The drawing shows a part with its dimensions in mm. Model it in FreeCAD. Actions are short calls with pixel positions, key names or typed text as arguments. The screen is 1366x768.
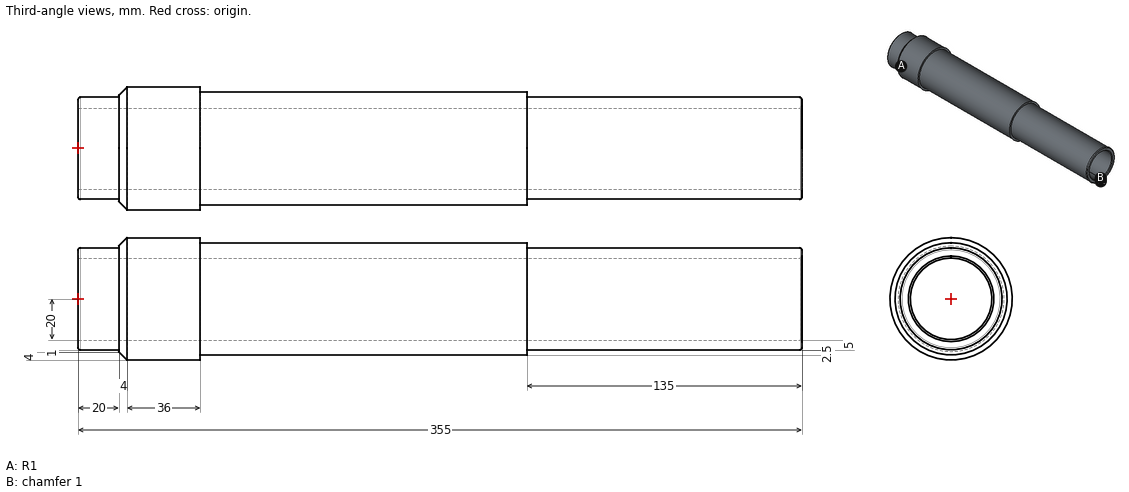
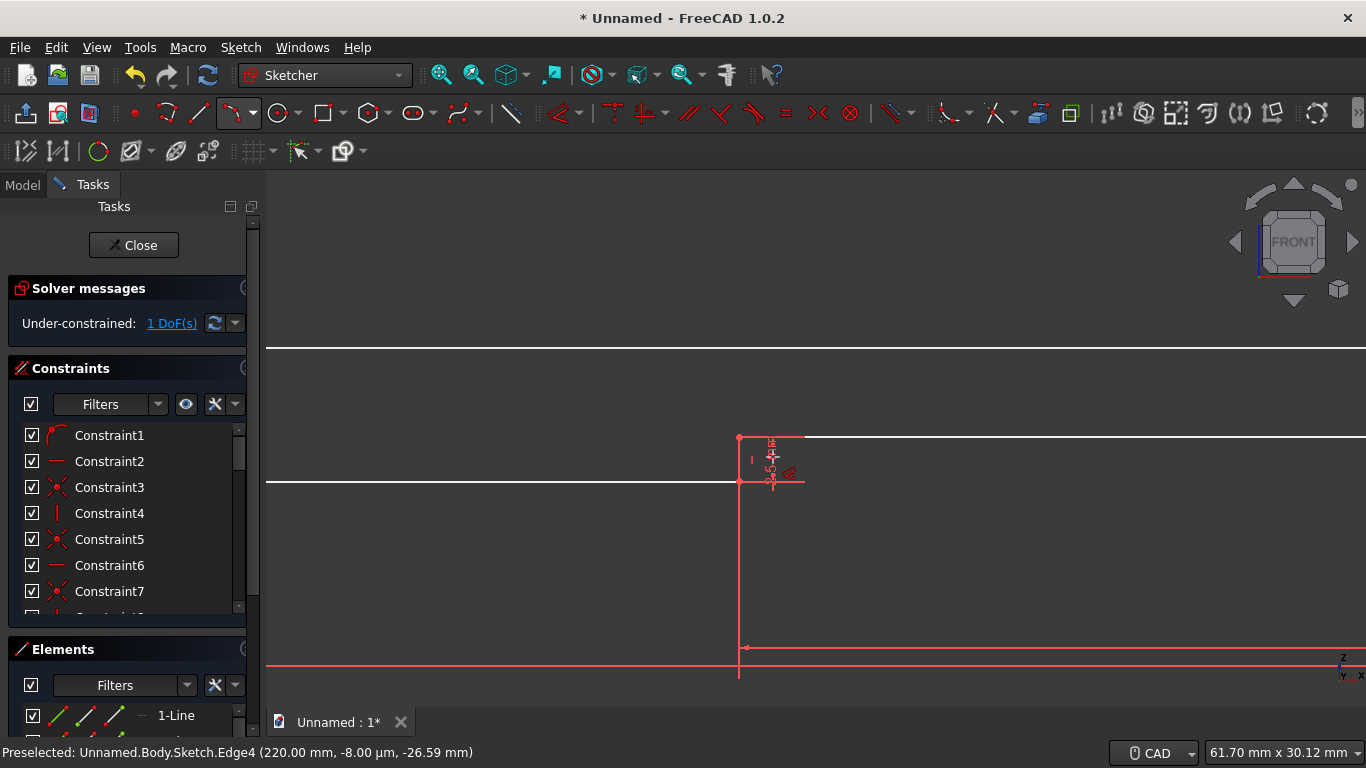
scroll(843, 462, down, 11)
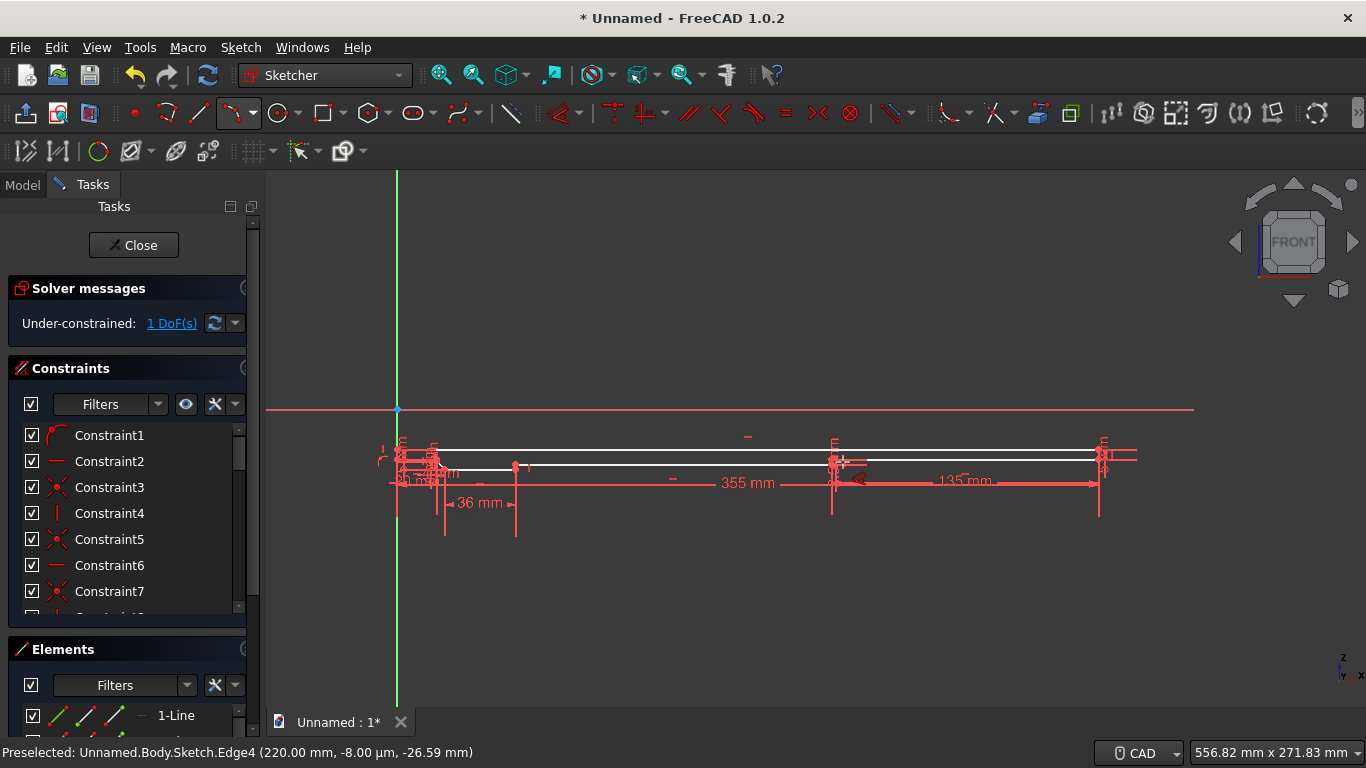
scroll(397, 450, up, 2)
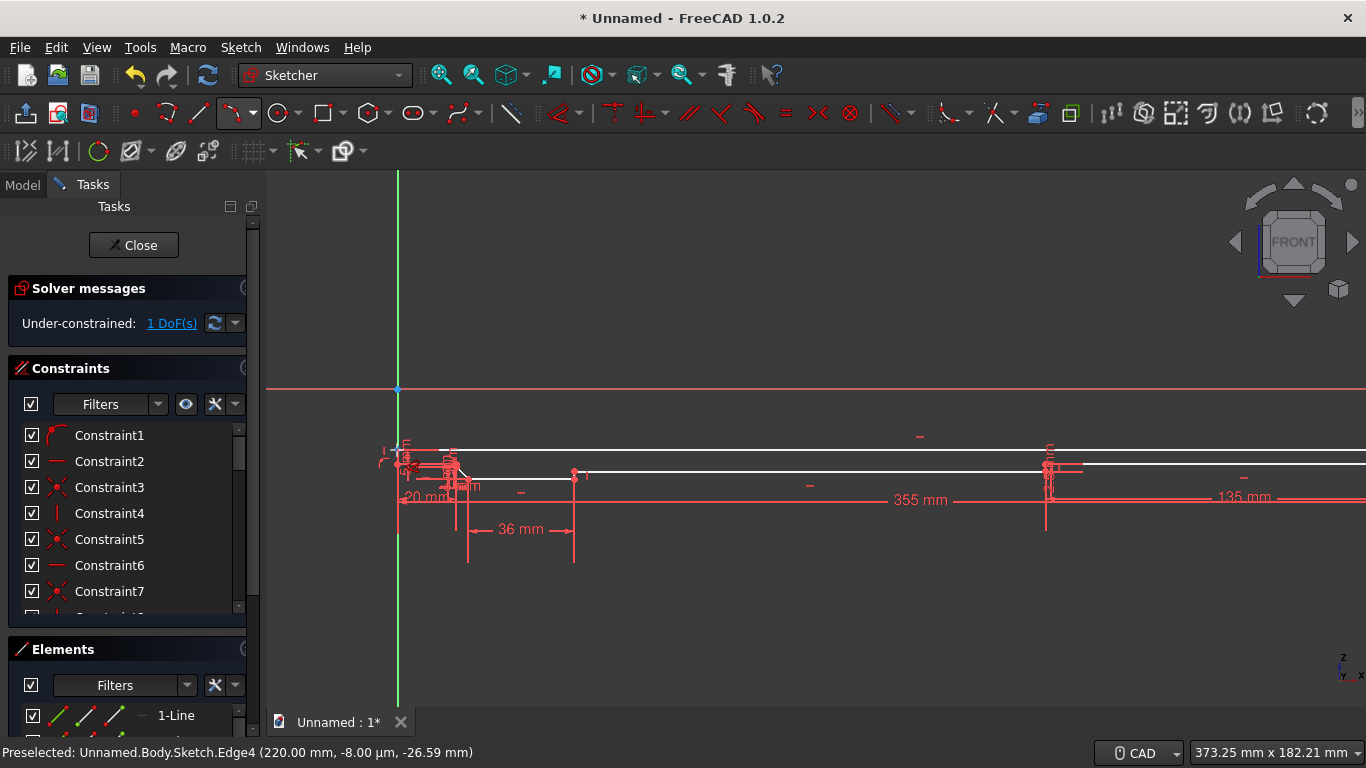
click(398, 450)
click(364, 419)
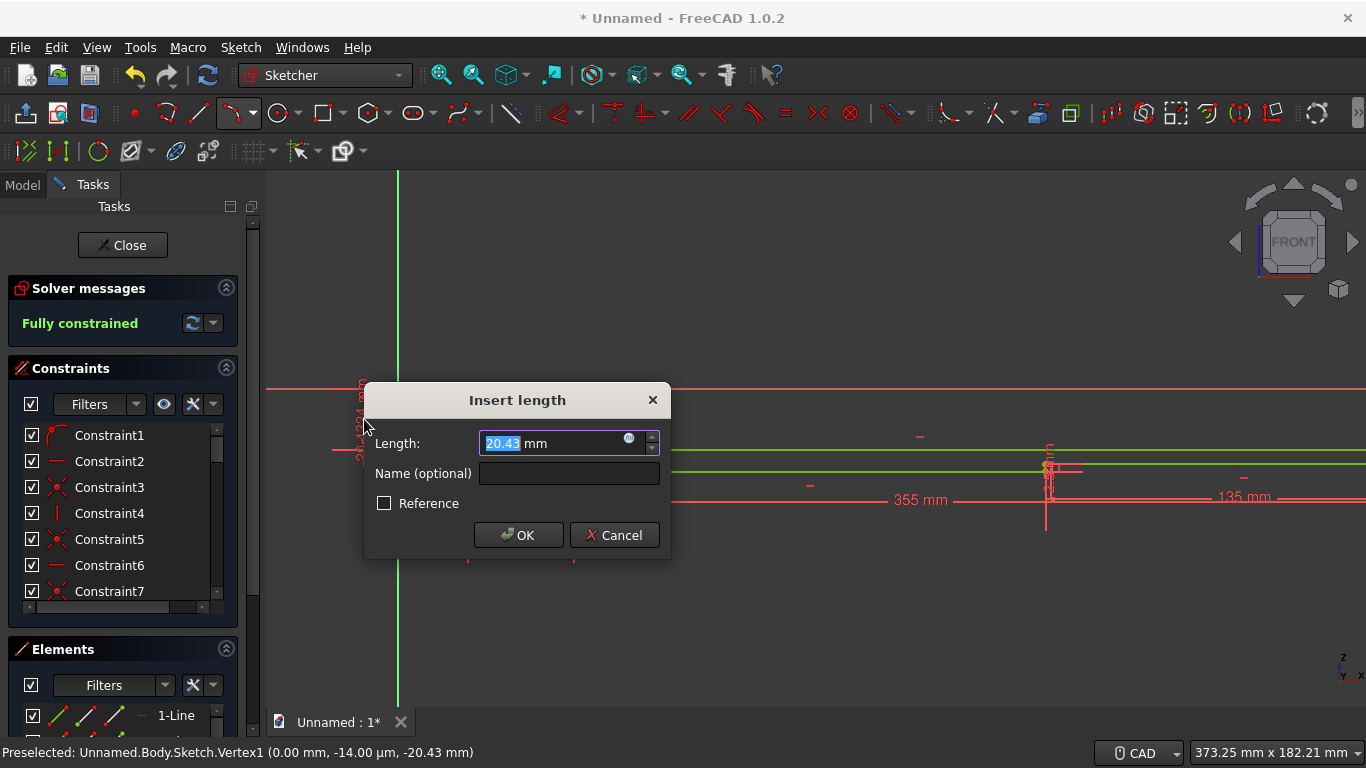
text(20)
key(Return)
key(Escape)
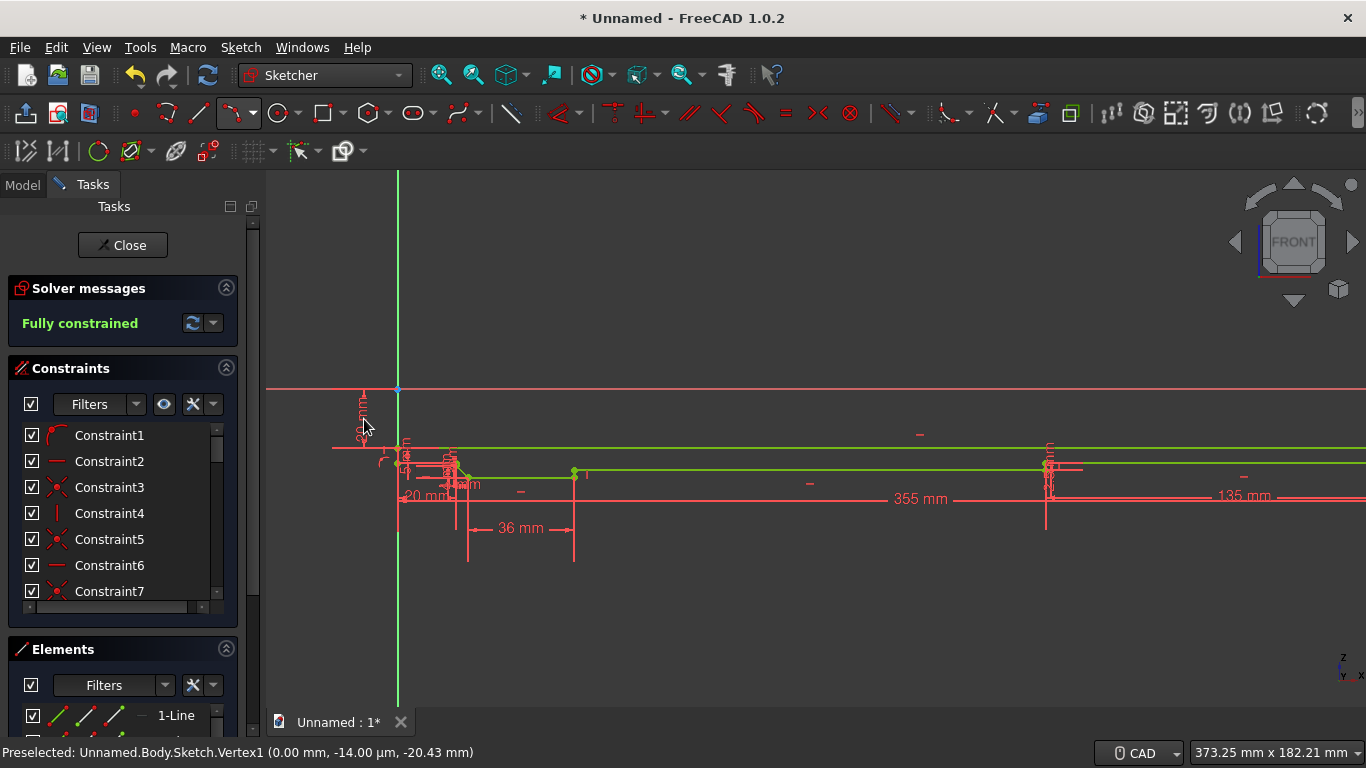
click(123, 245)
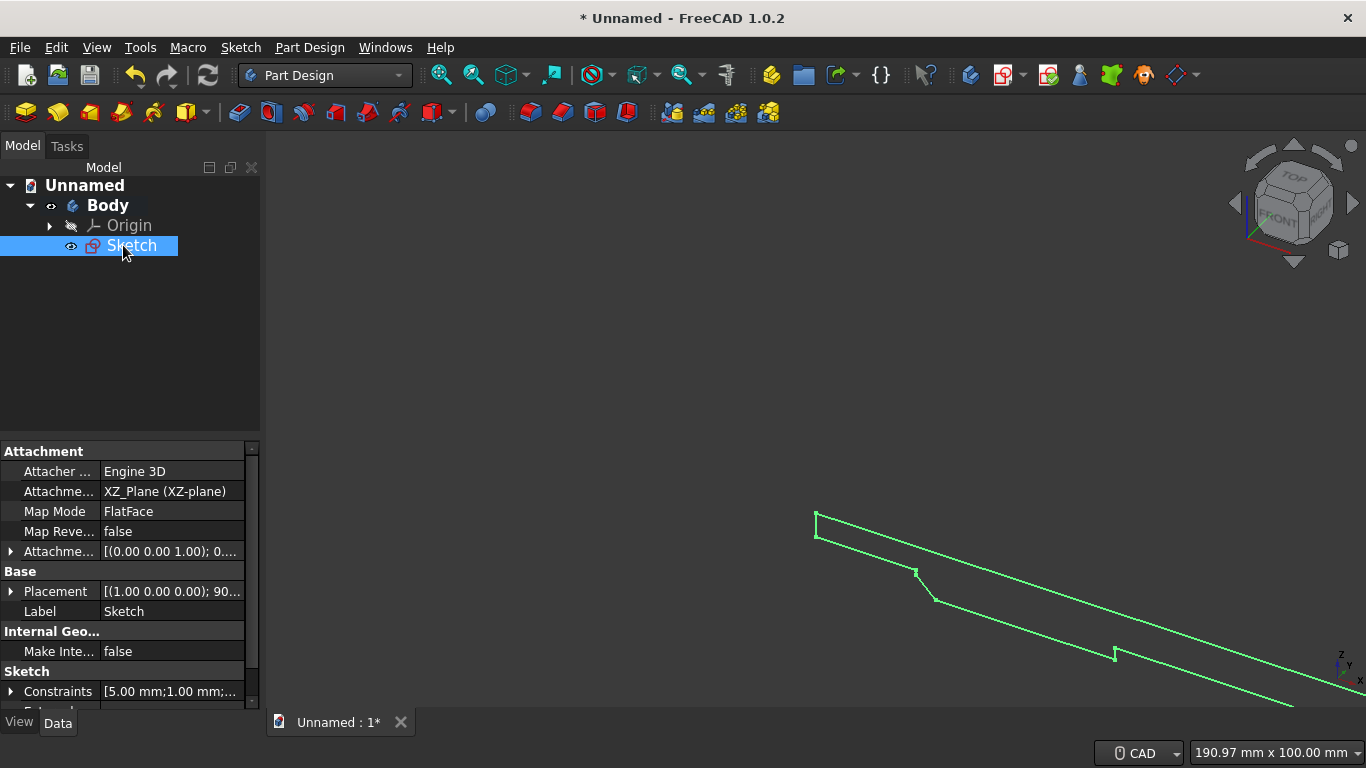
click(58, 112)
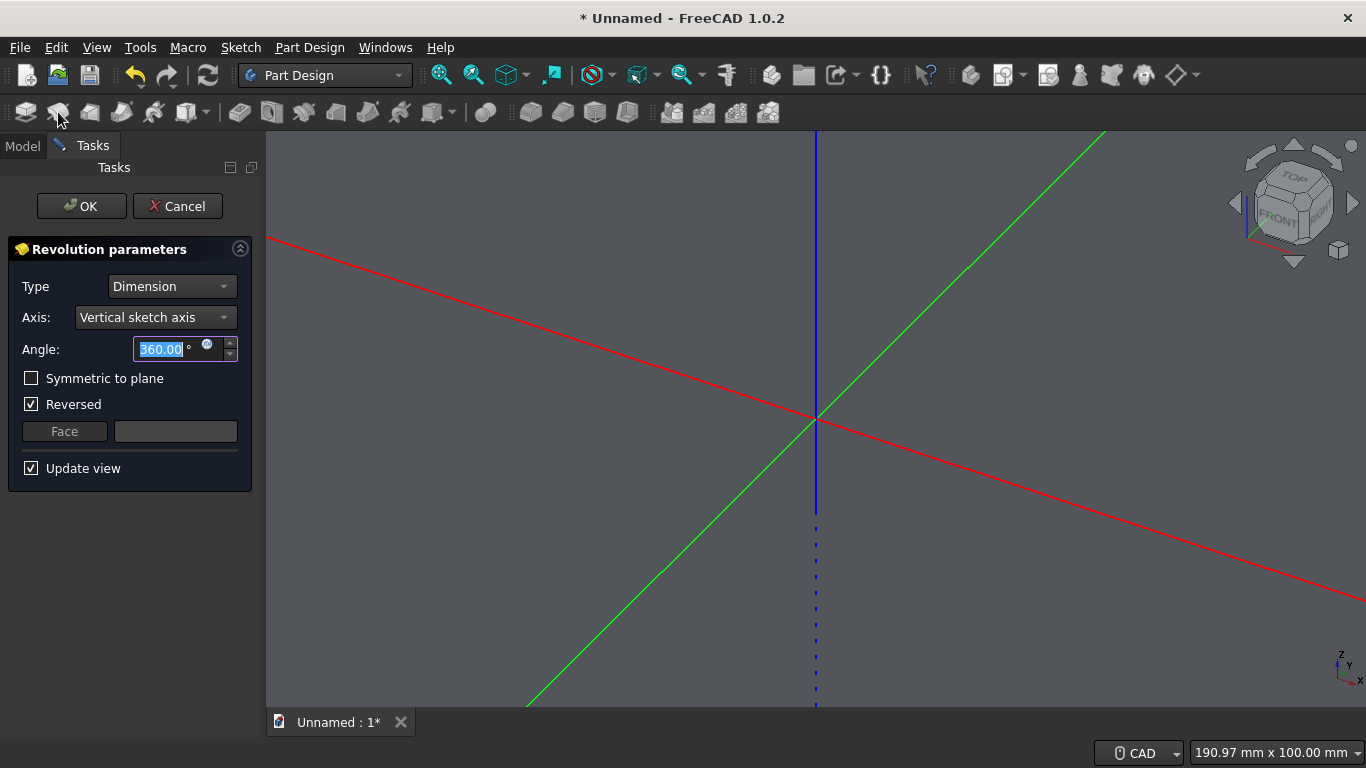
click(156, 318)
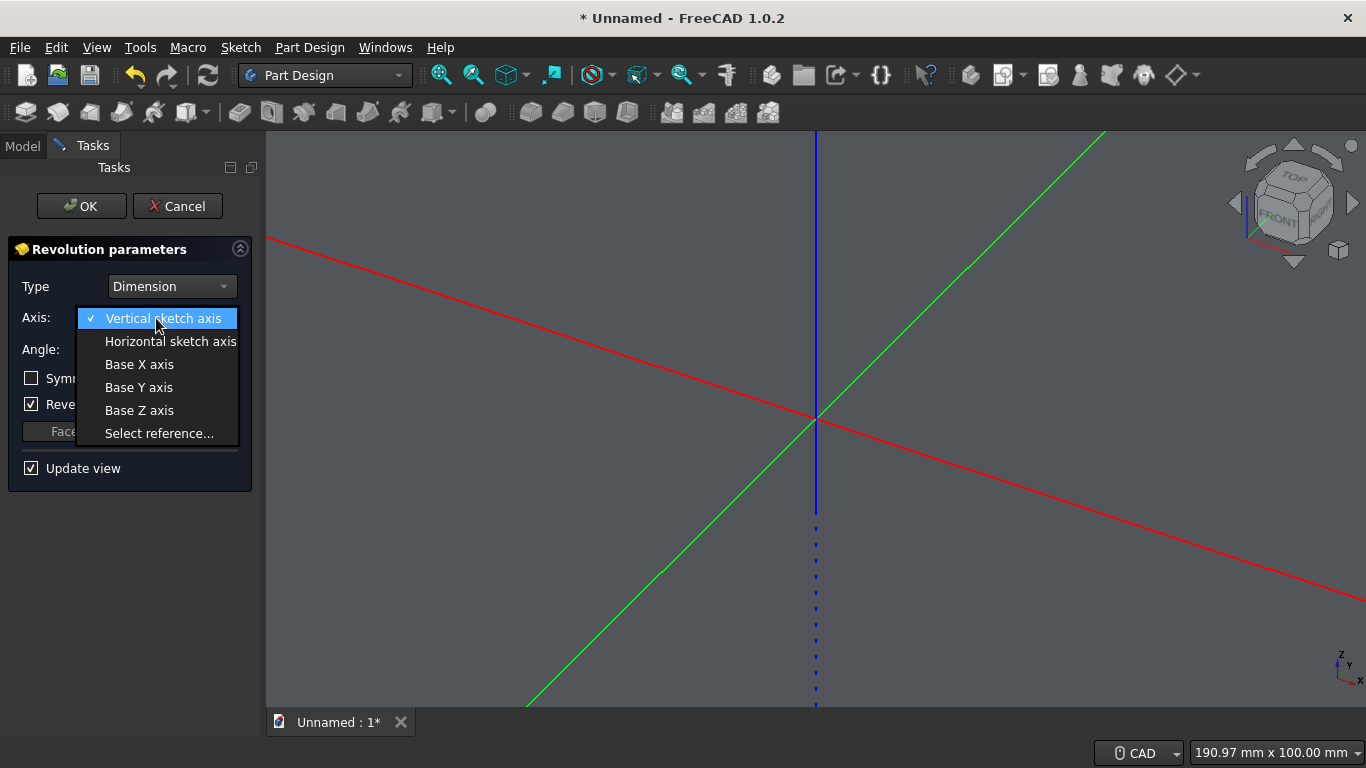
click(156, 342)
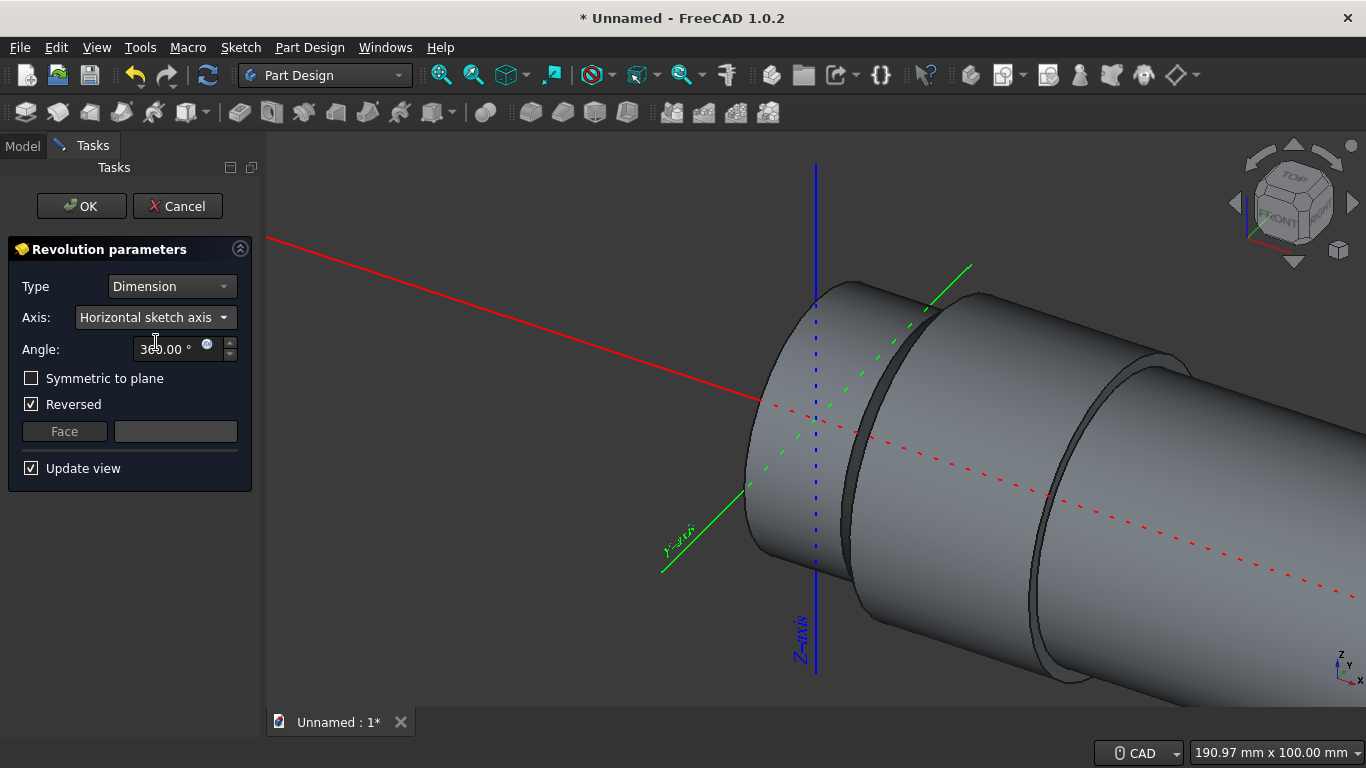
click(82, 206)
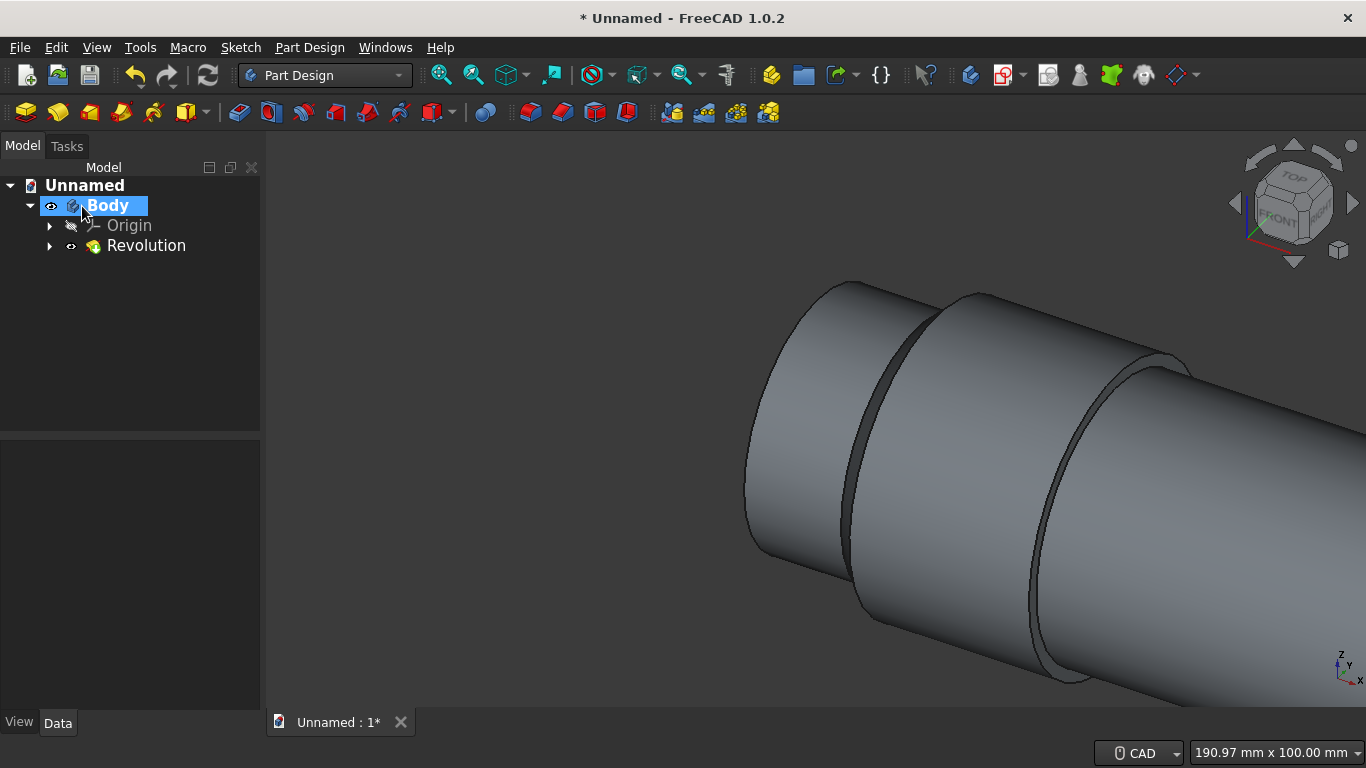
key(v)
key(f)